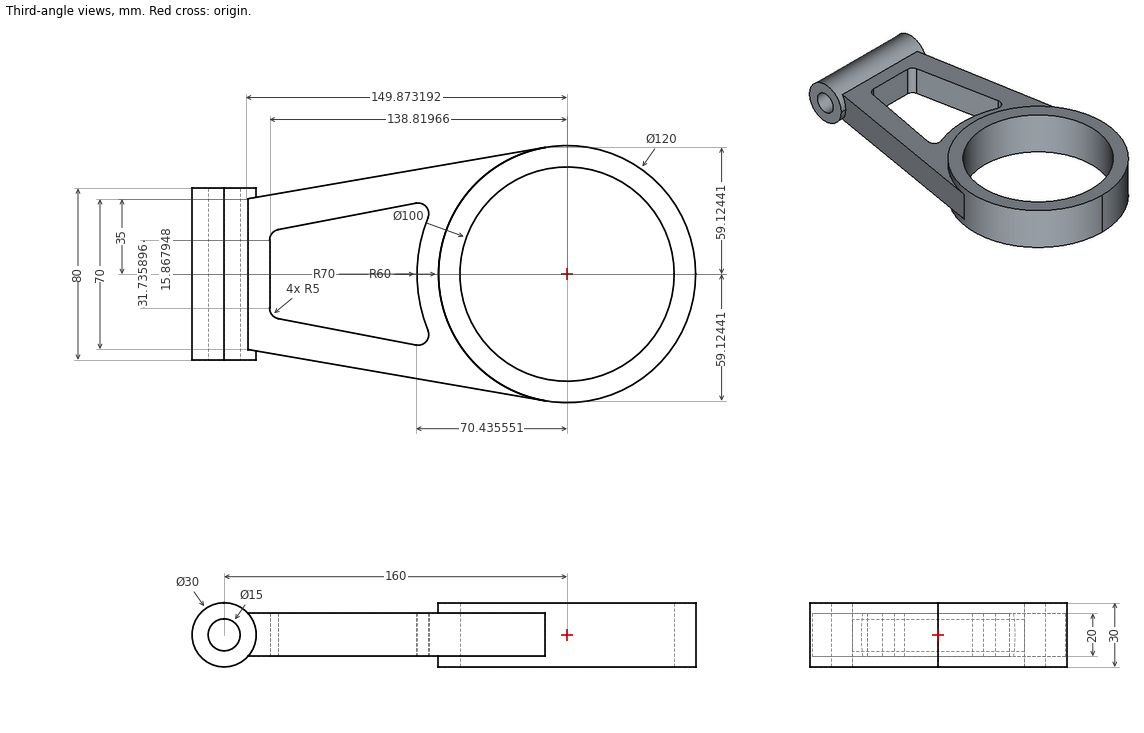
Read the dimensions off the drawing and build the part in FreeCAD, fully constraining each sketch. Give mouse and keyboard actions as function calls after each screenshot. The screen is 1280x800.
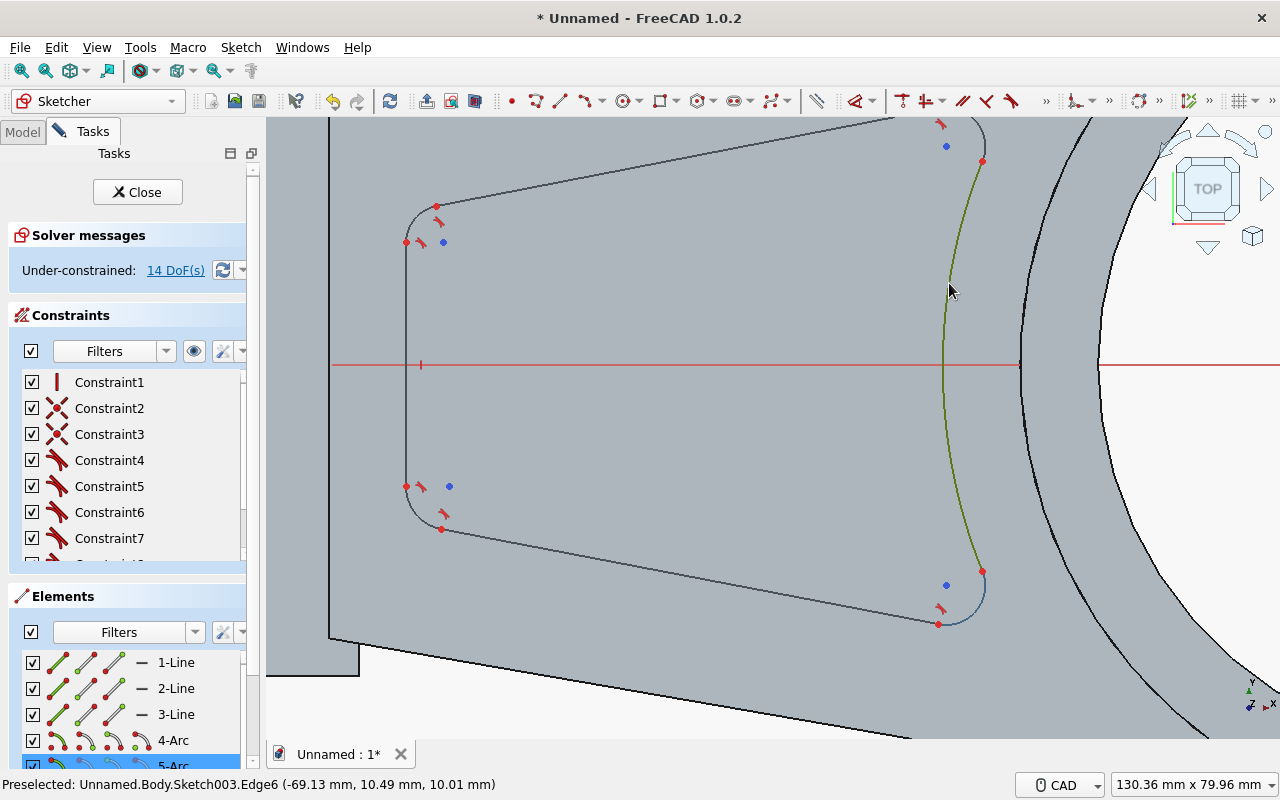
click(1012, 102)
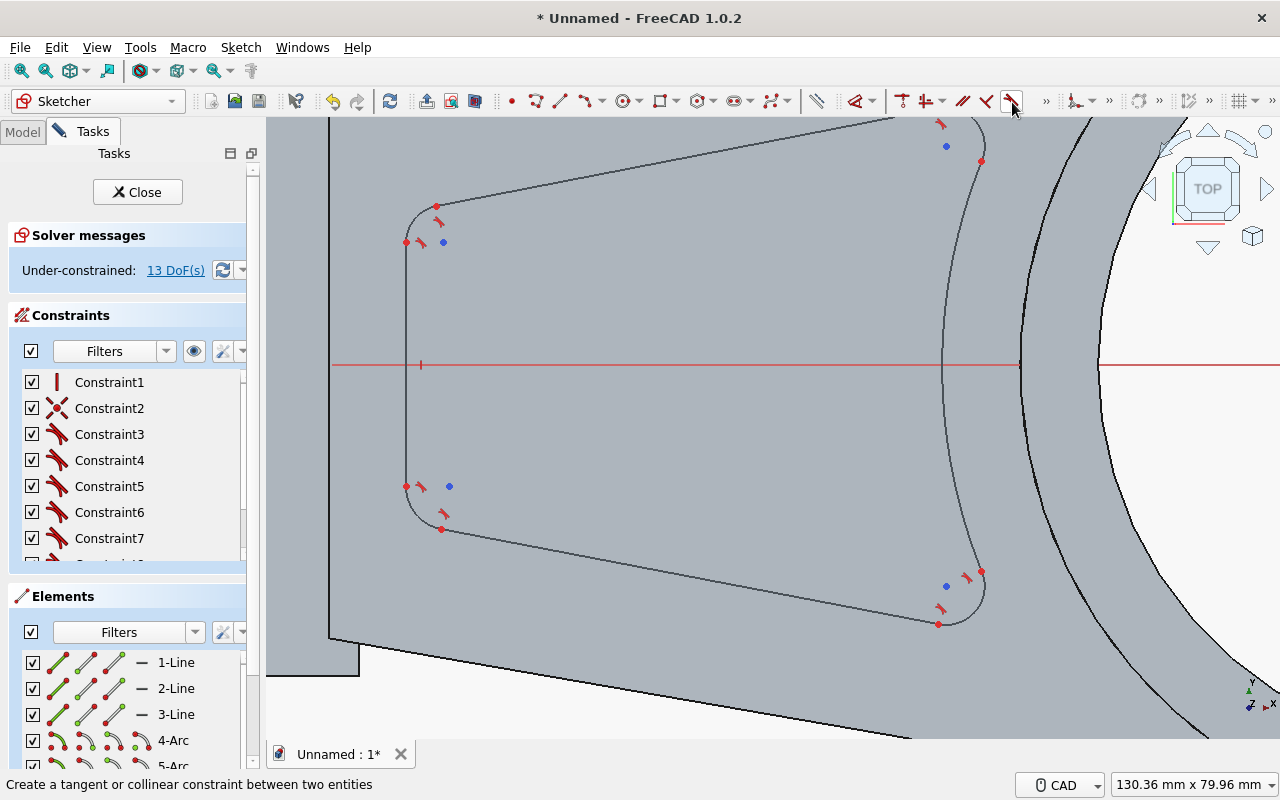
click(949, 283)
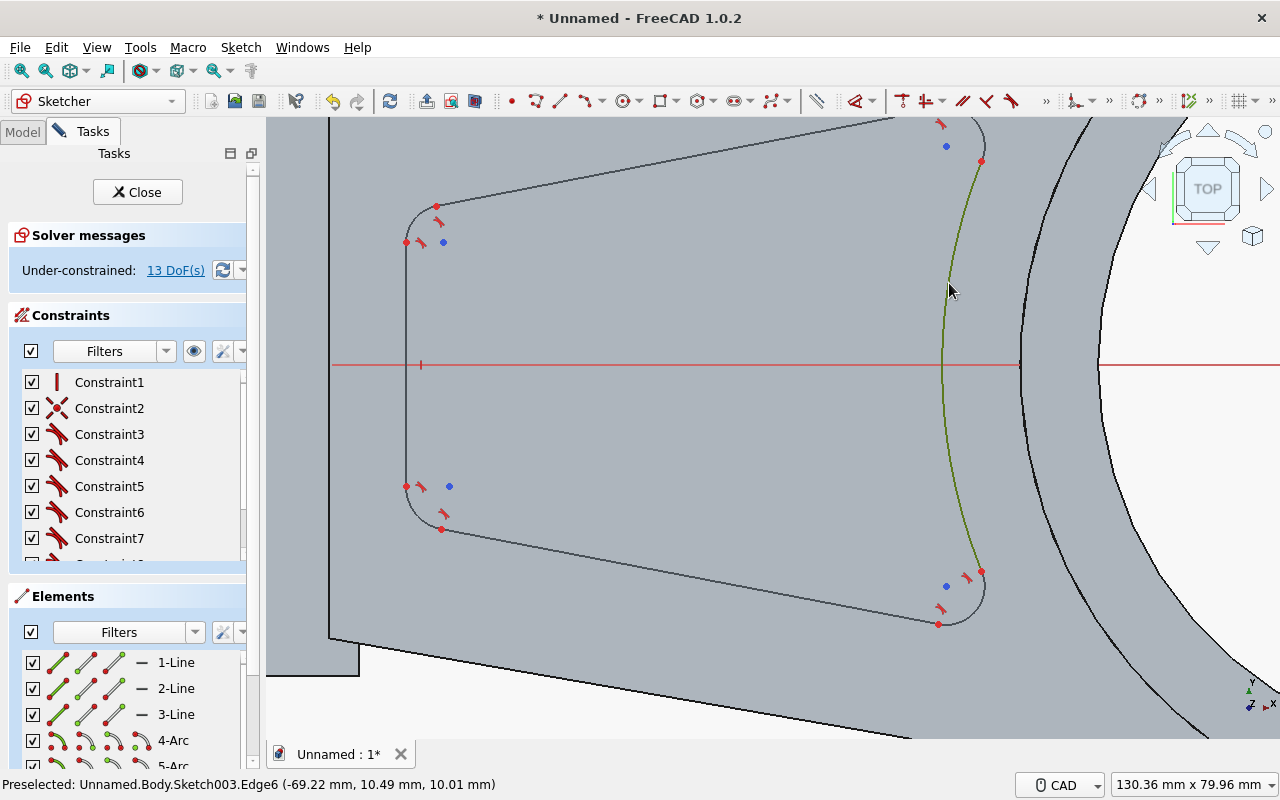
click(985, 145)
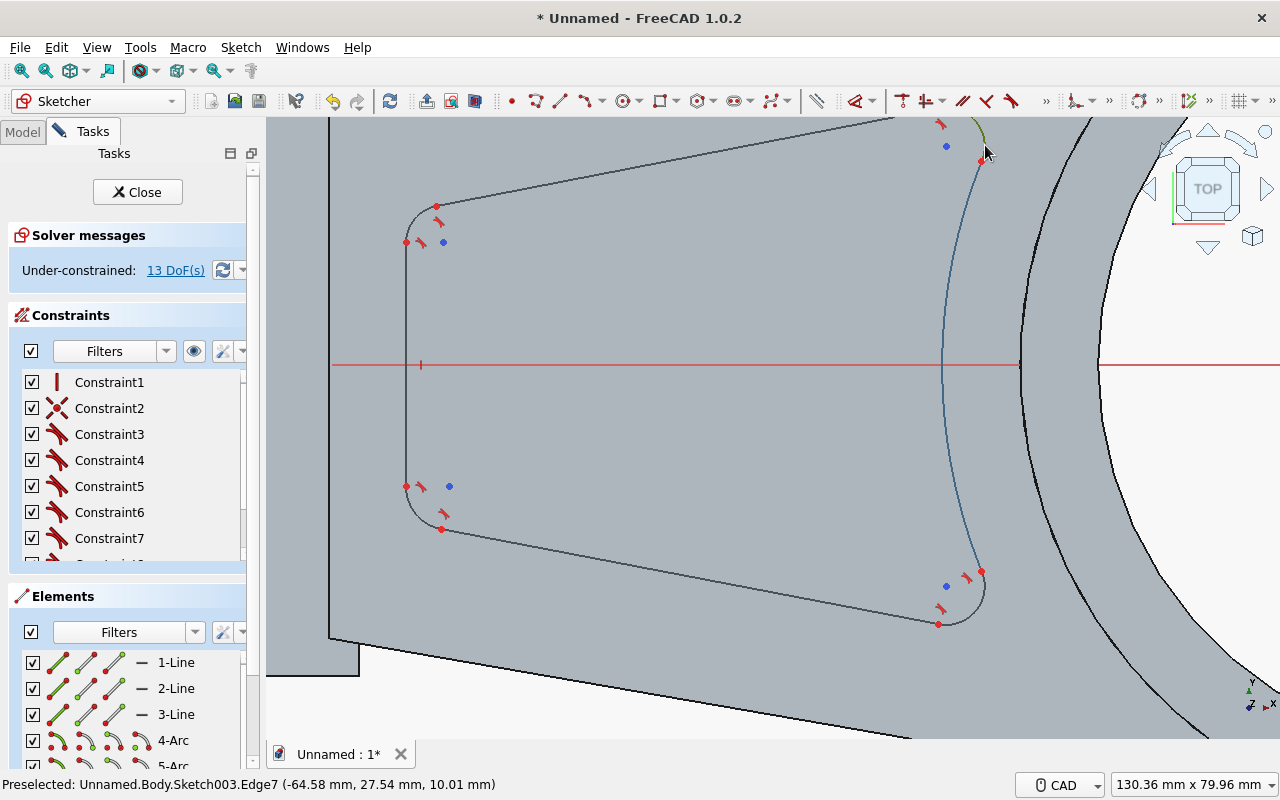
click(1012, 102)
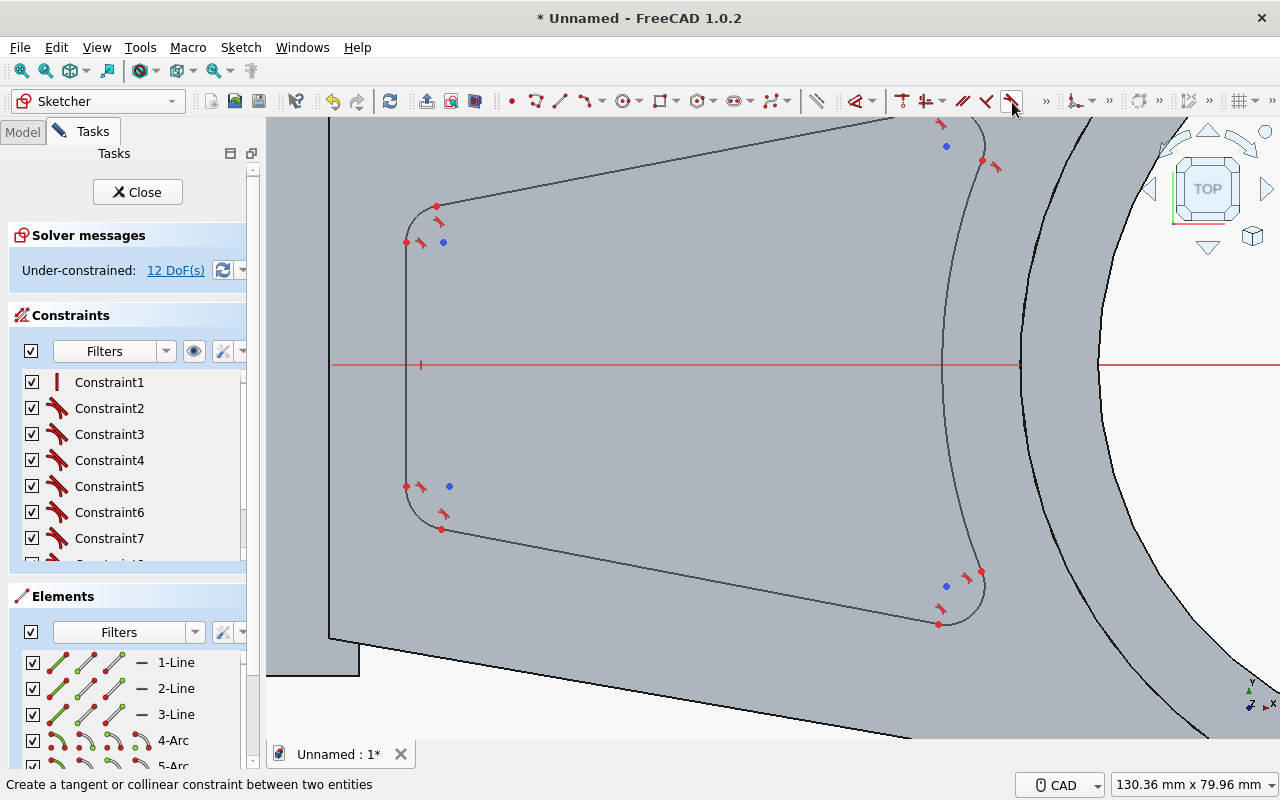
scroll(409, 505, down, 3)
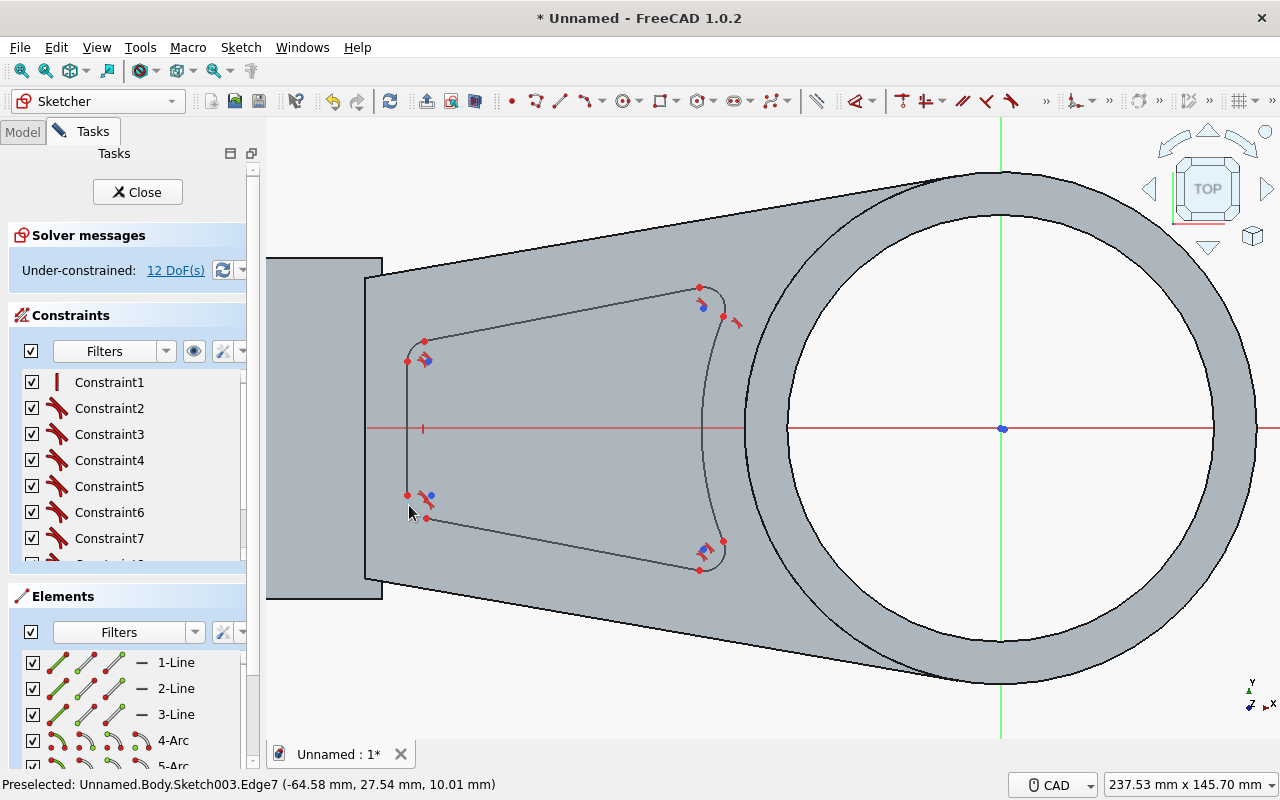
scroll(1002, 429, up, 4)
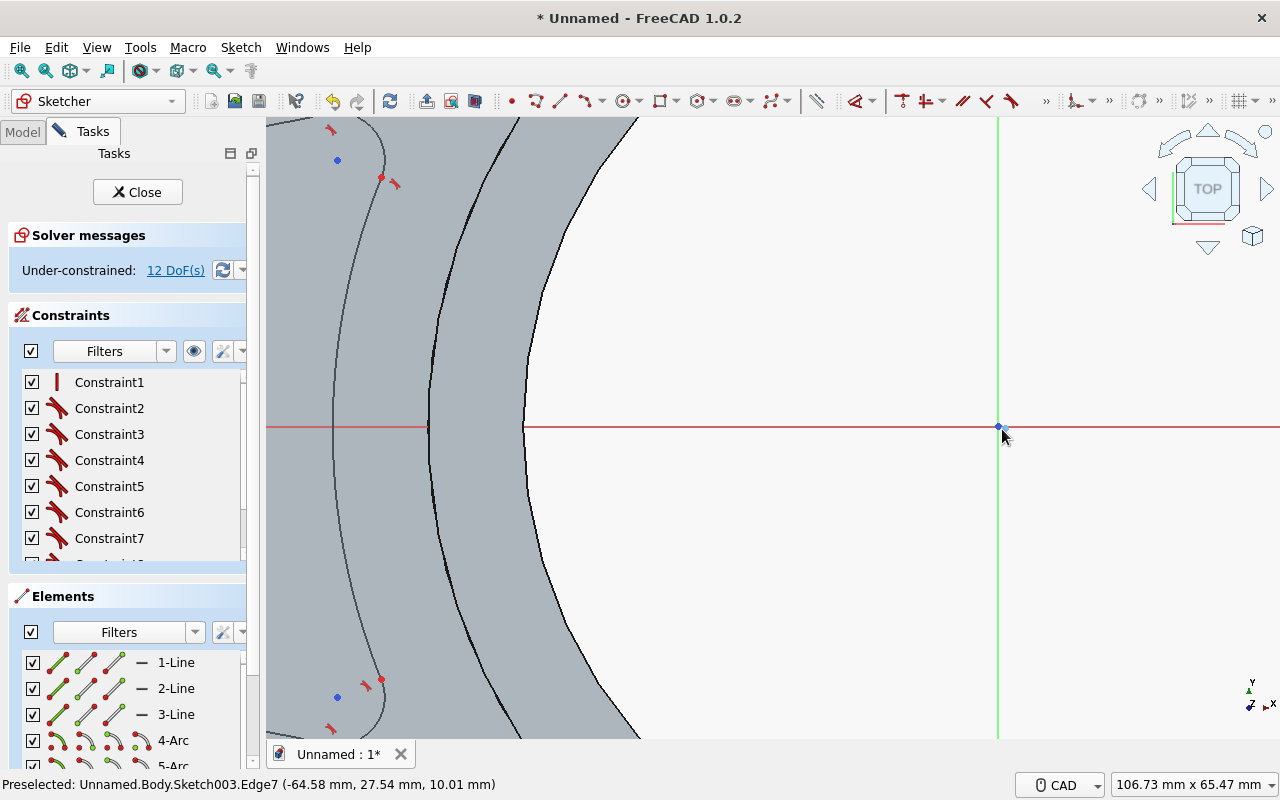
drag(988, 417, 1016, 439)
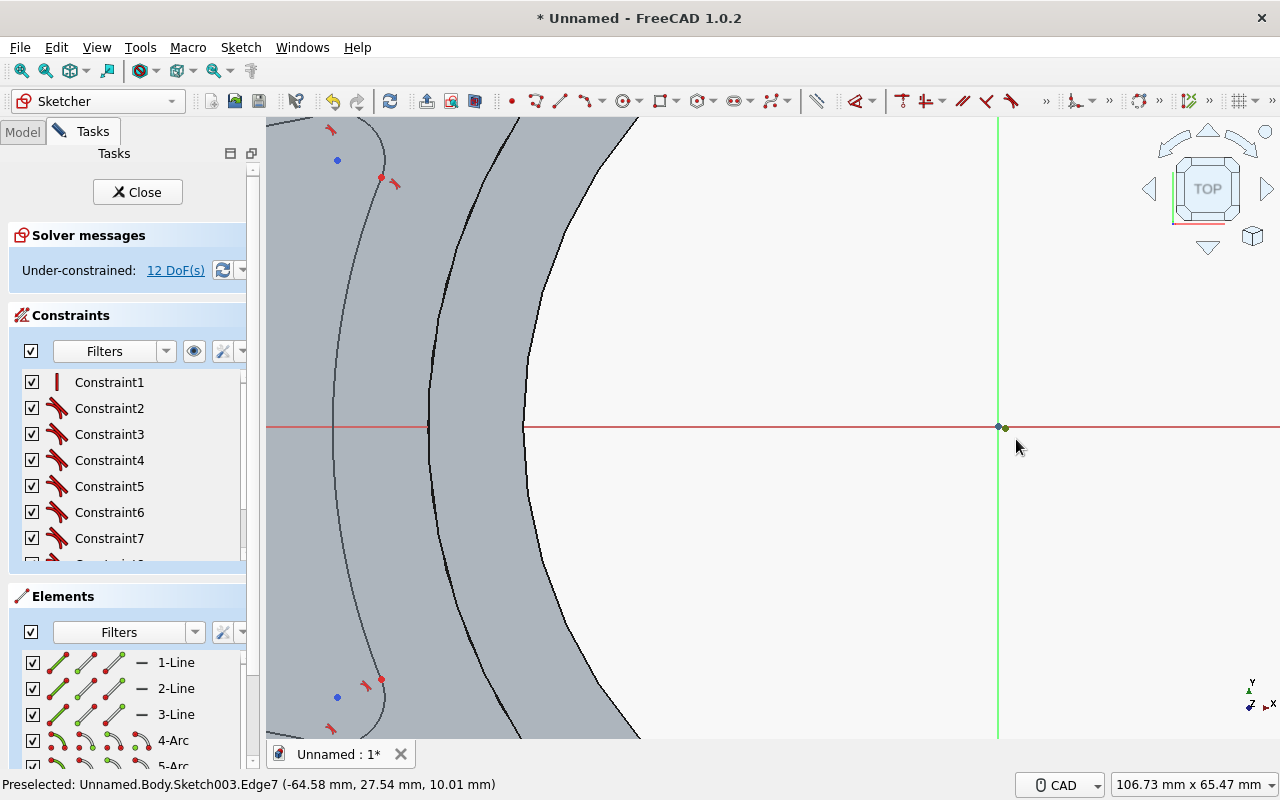
click(902, 102)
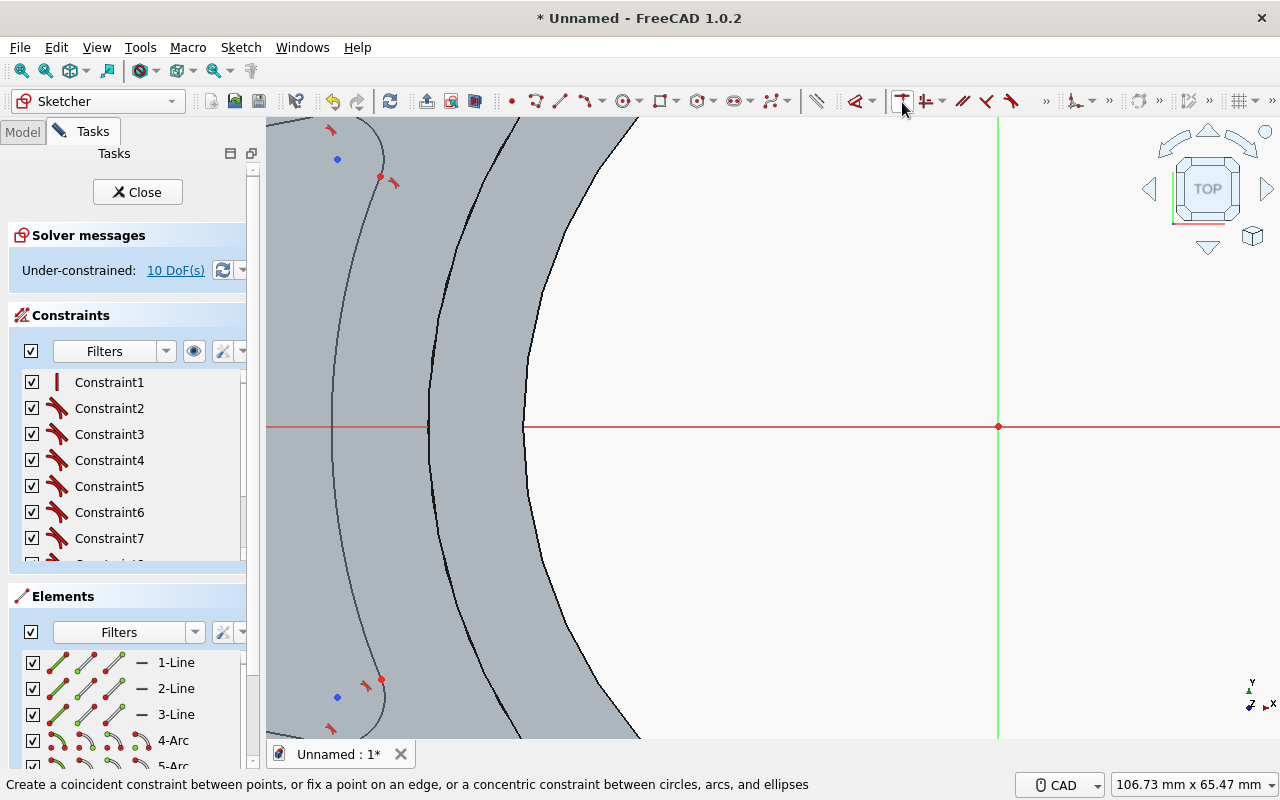
scroll(1003, 429, down, 4)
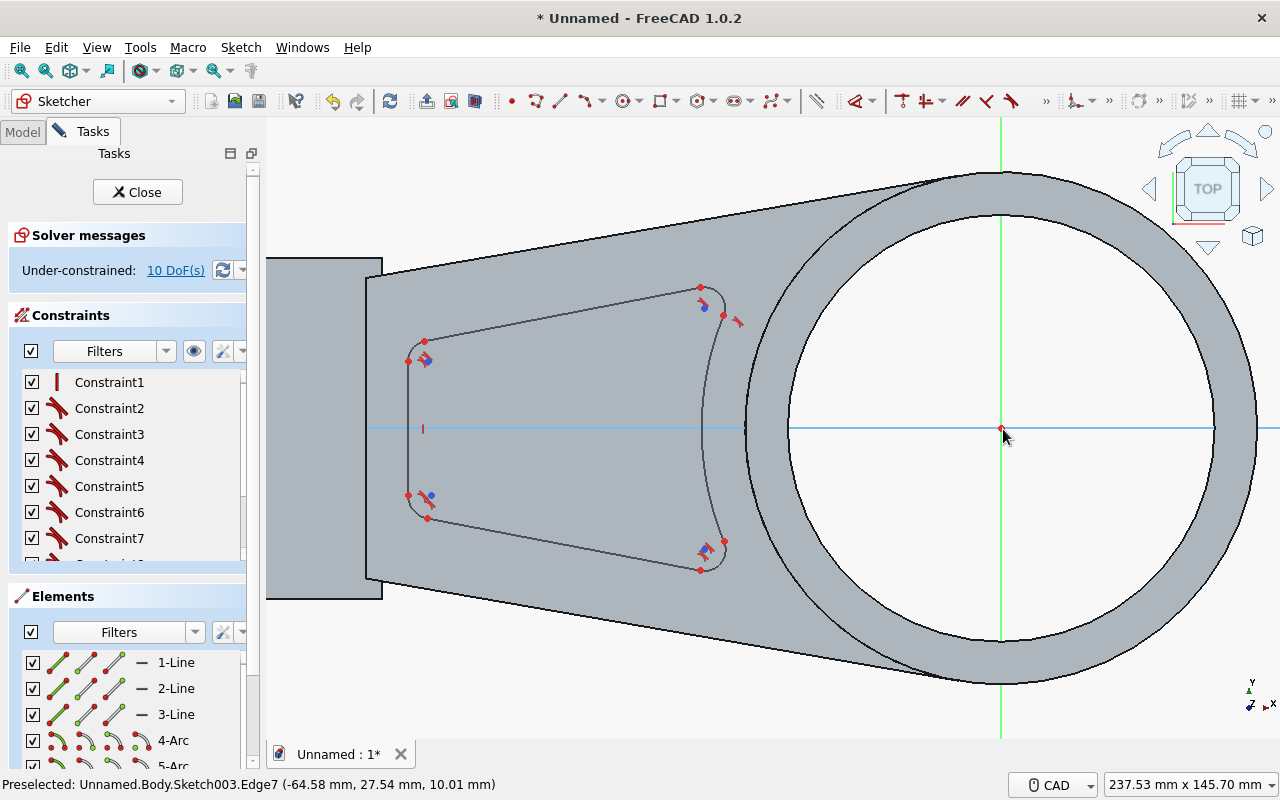
scroll(410, 505, up, 2)